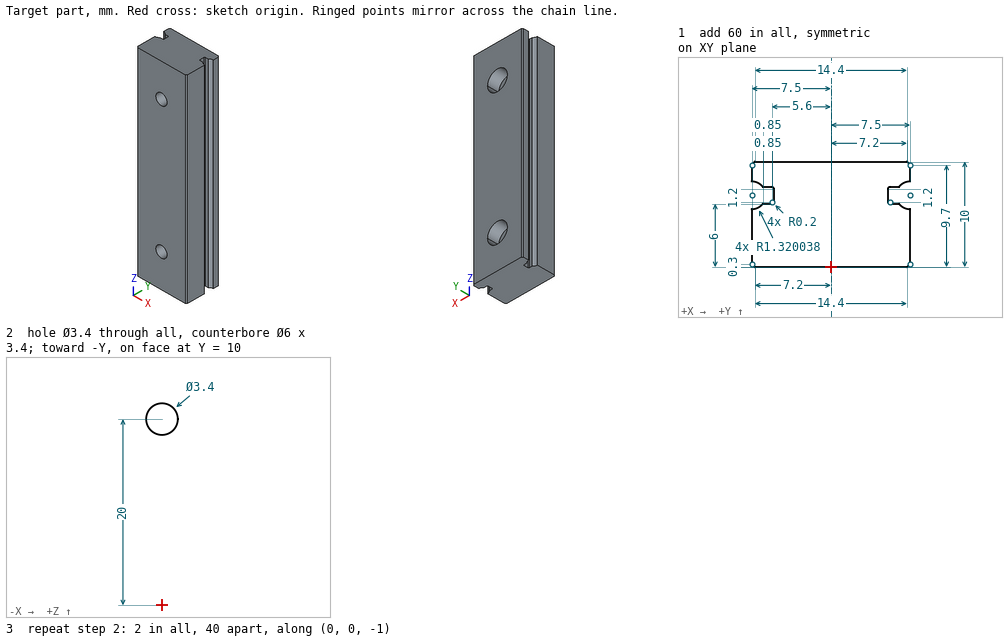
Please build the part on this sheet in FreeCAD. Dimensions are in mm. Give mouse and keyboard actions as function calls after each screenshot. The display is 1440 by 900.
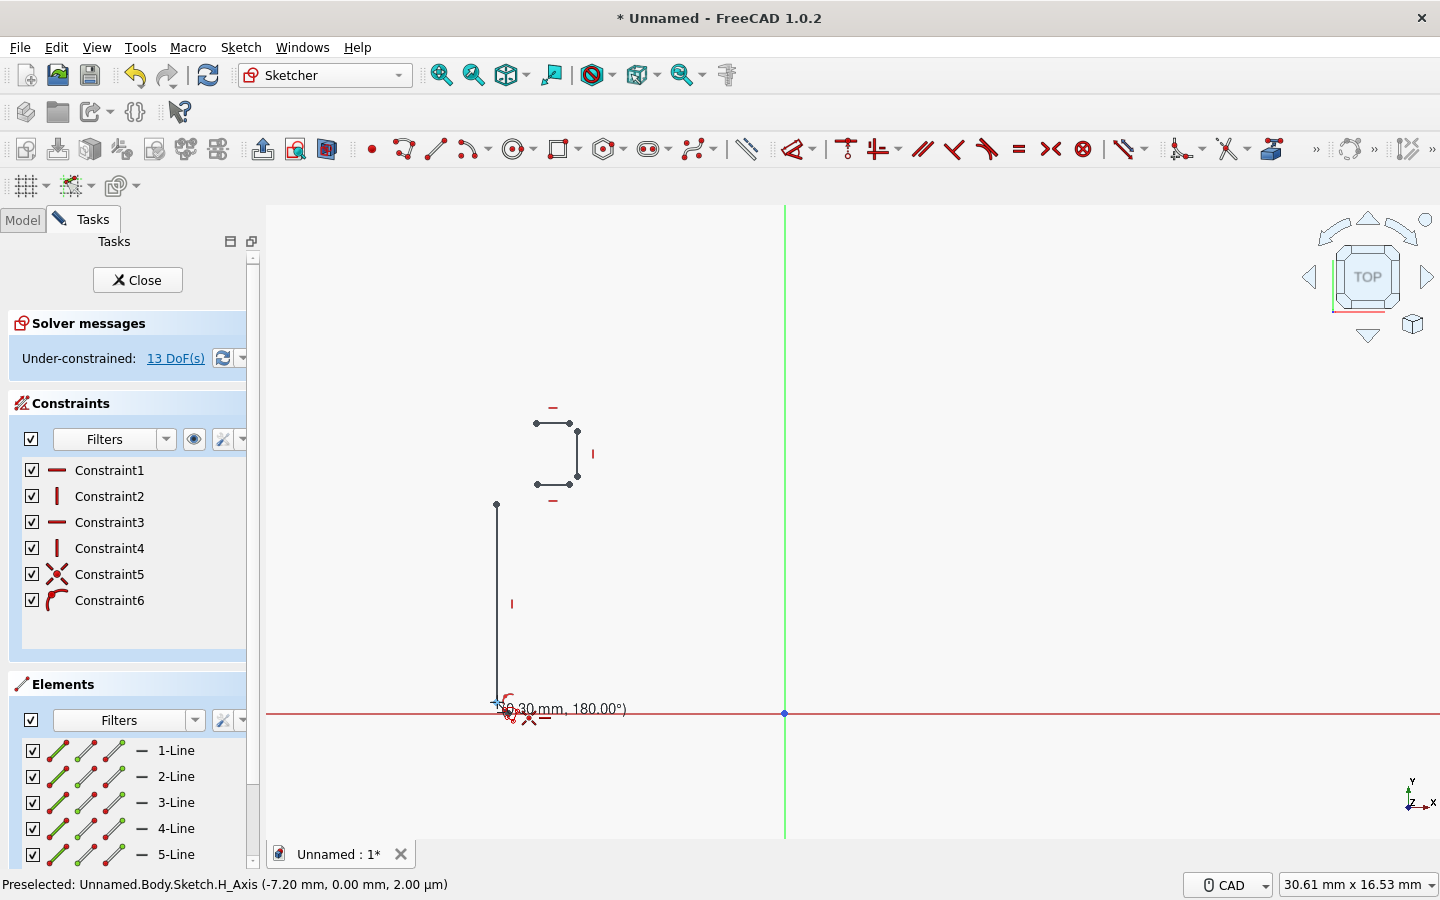
click(1061, 705)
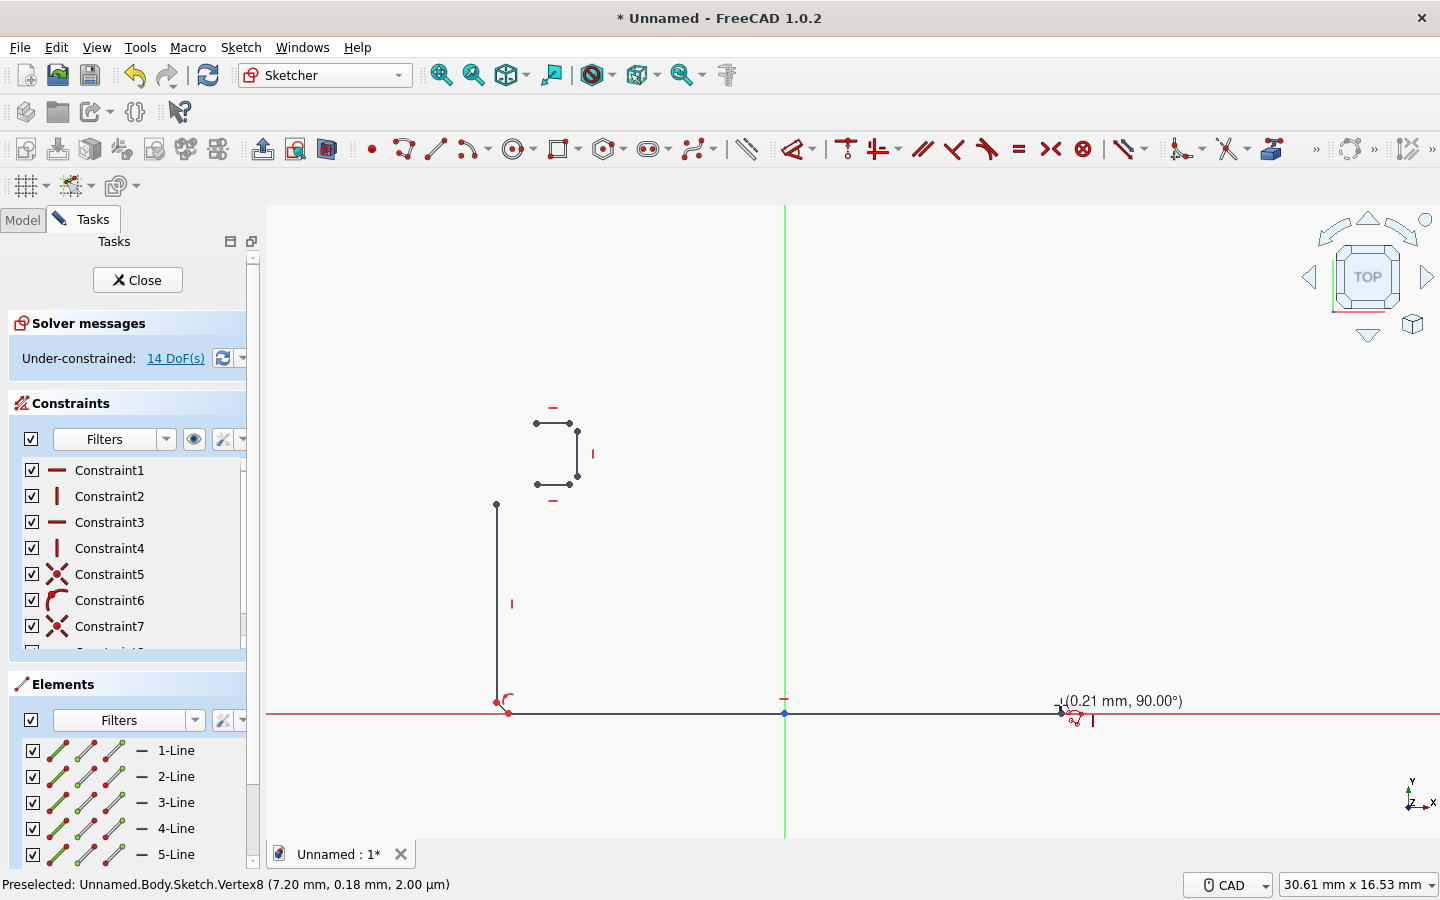
scroll(1072, 702, up, 2)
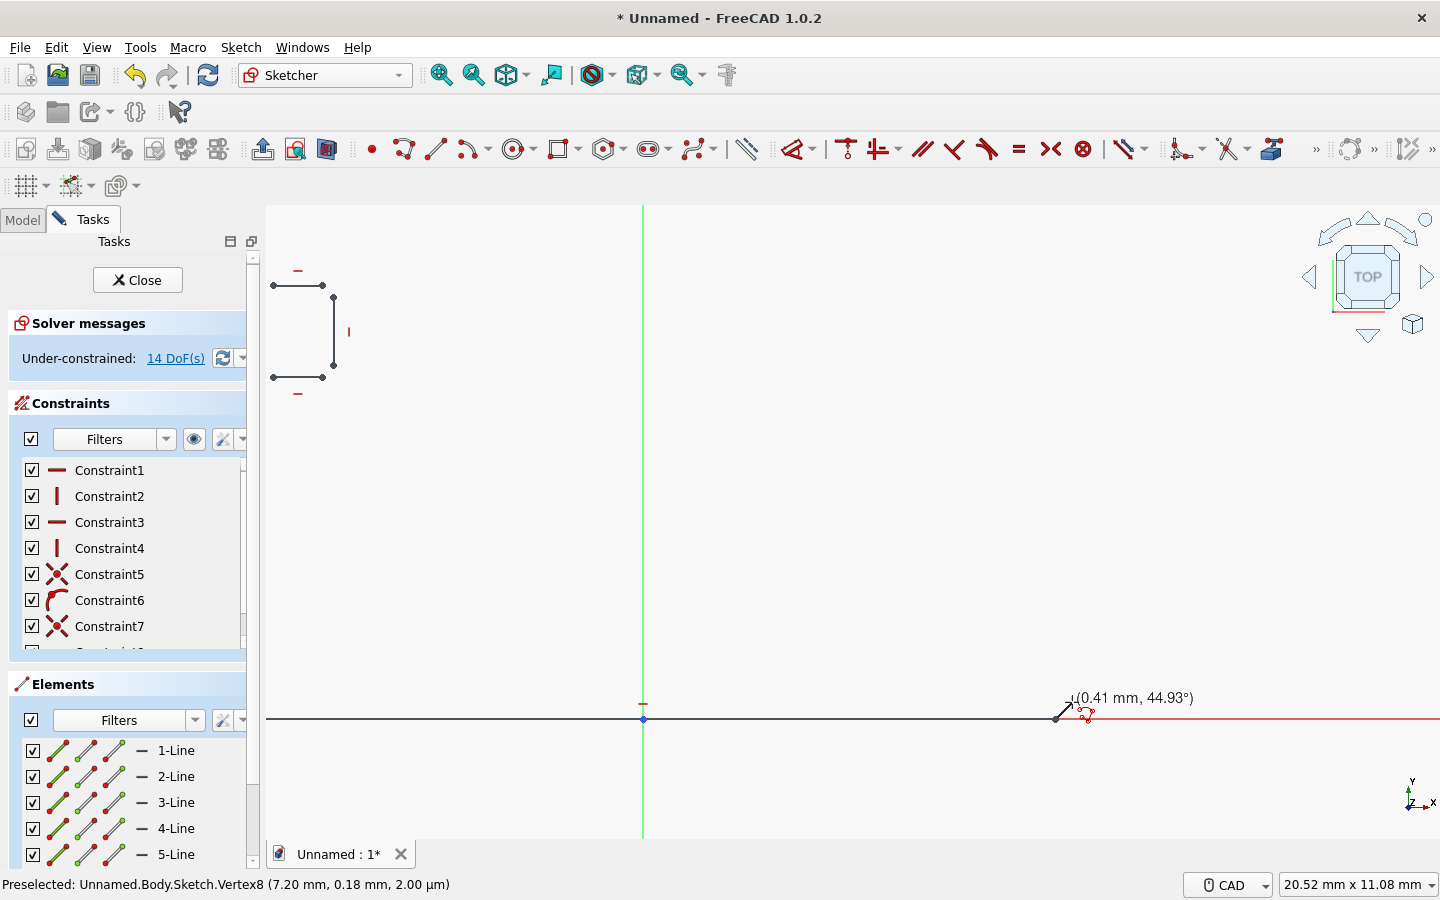
click(1072, 702)
click(1072, 406)
right_click(1072, 406)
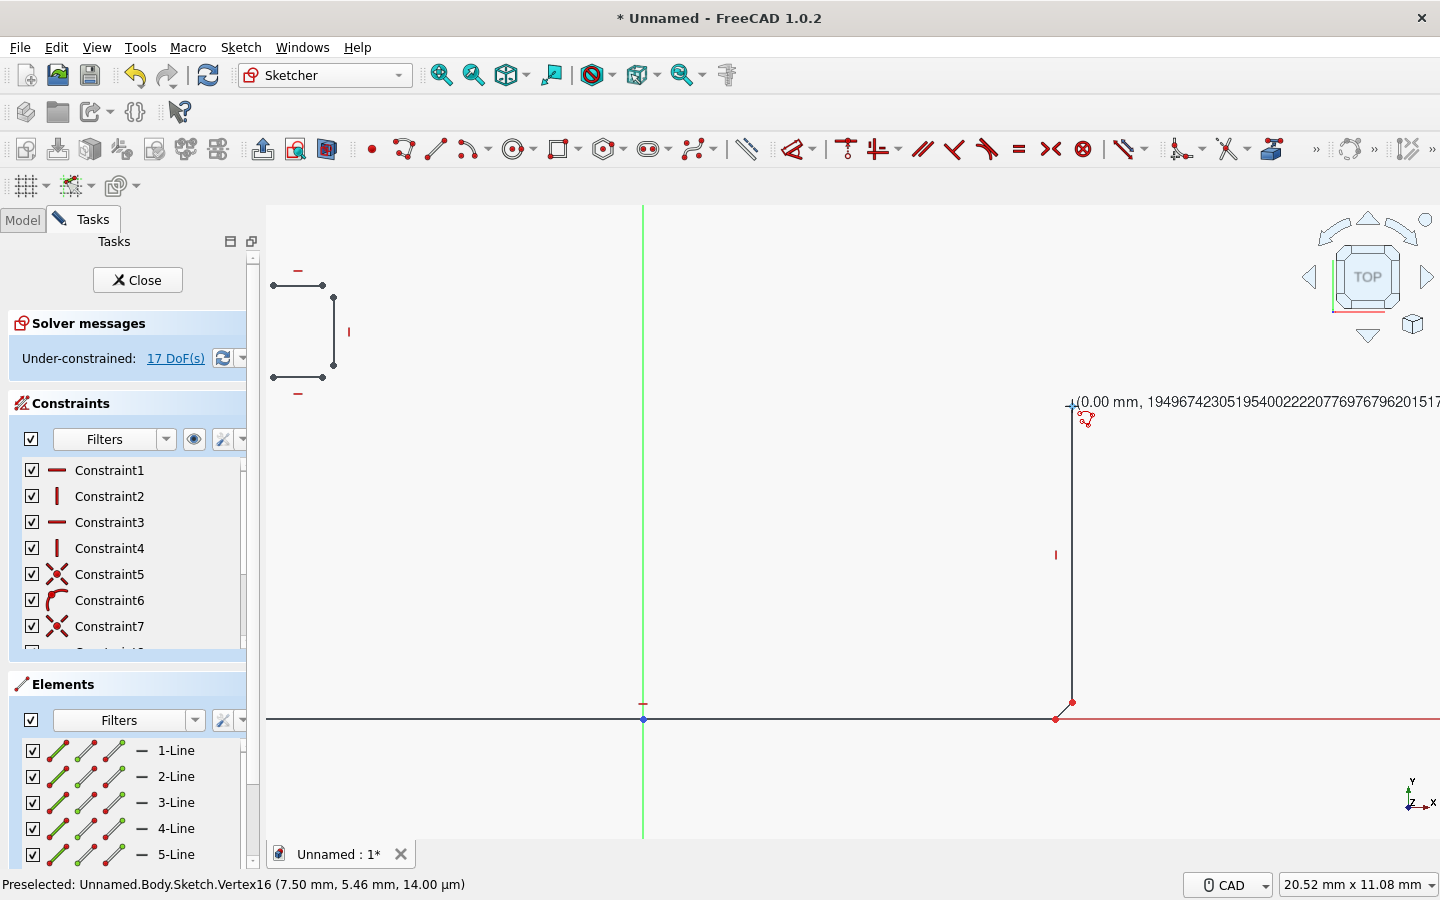
click(436, 150)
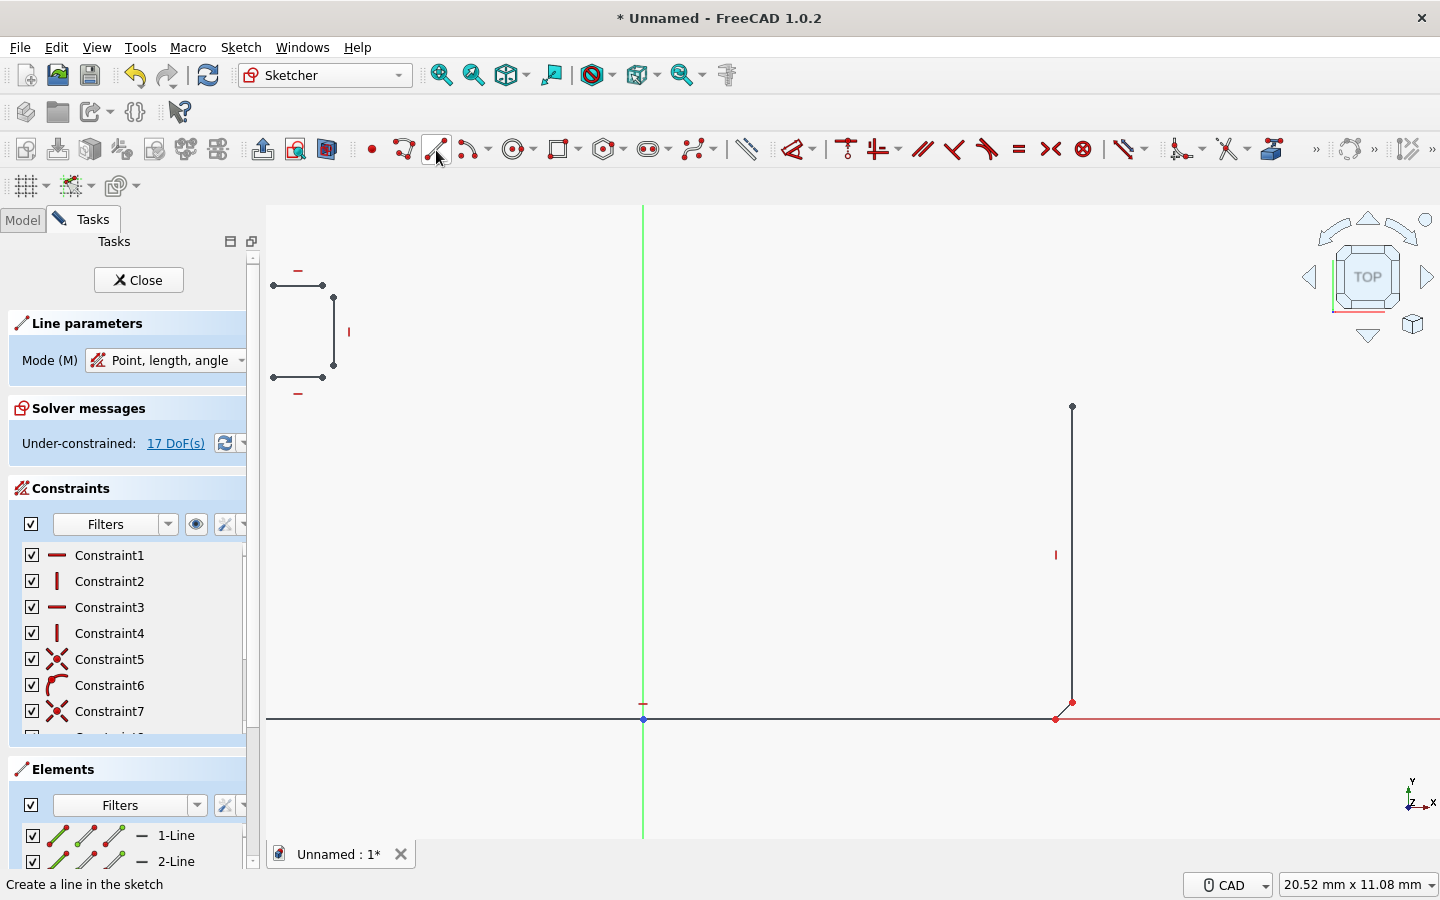
click(1012, 376)
click(963, 376)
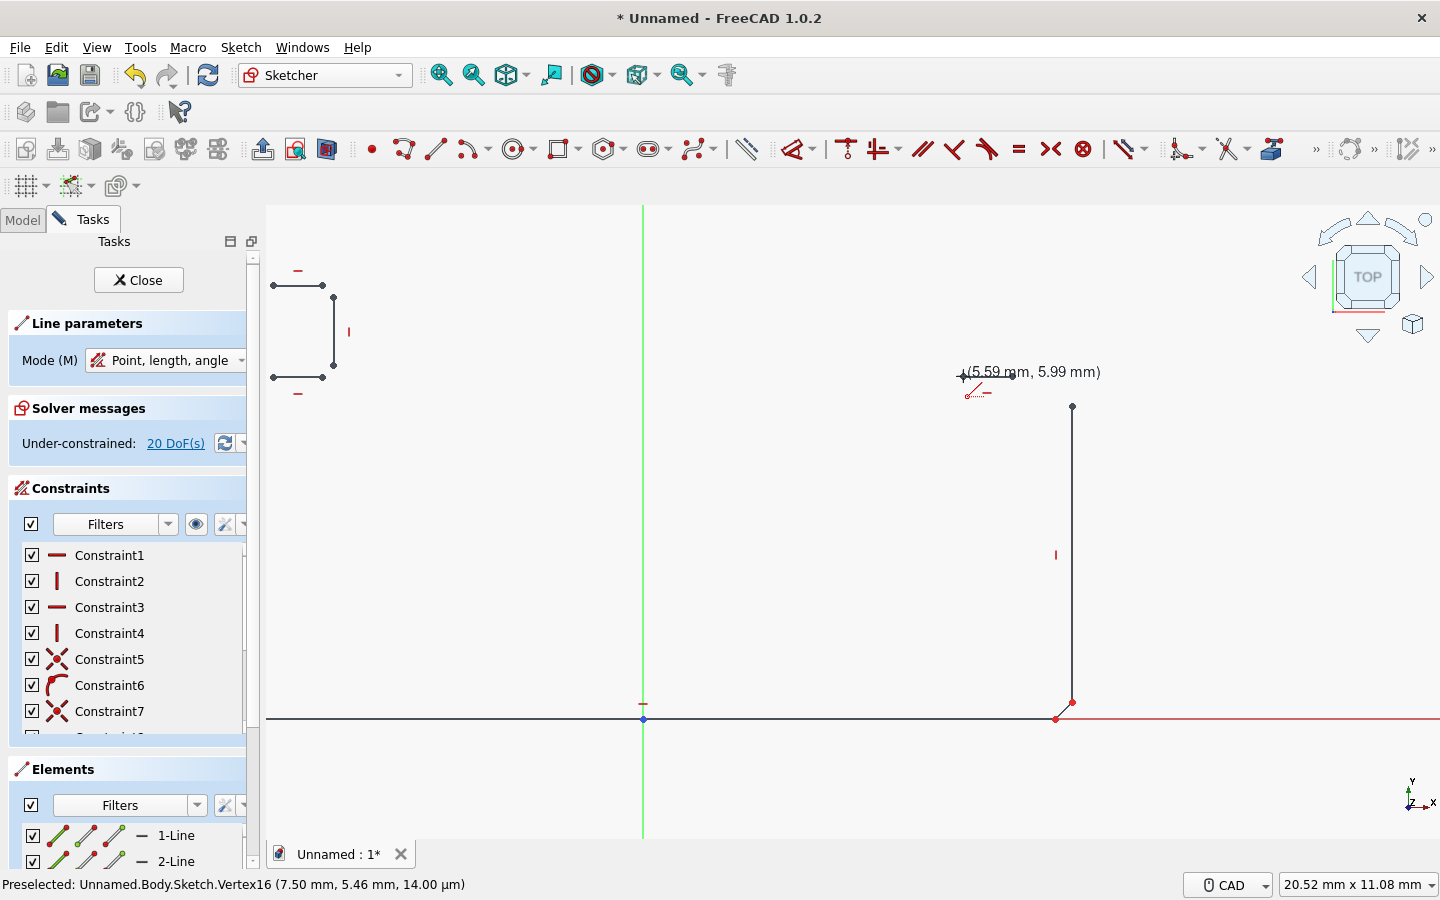
click(952, 365)
click(952, 296)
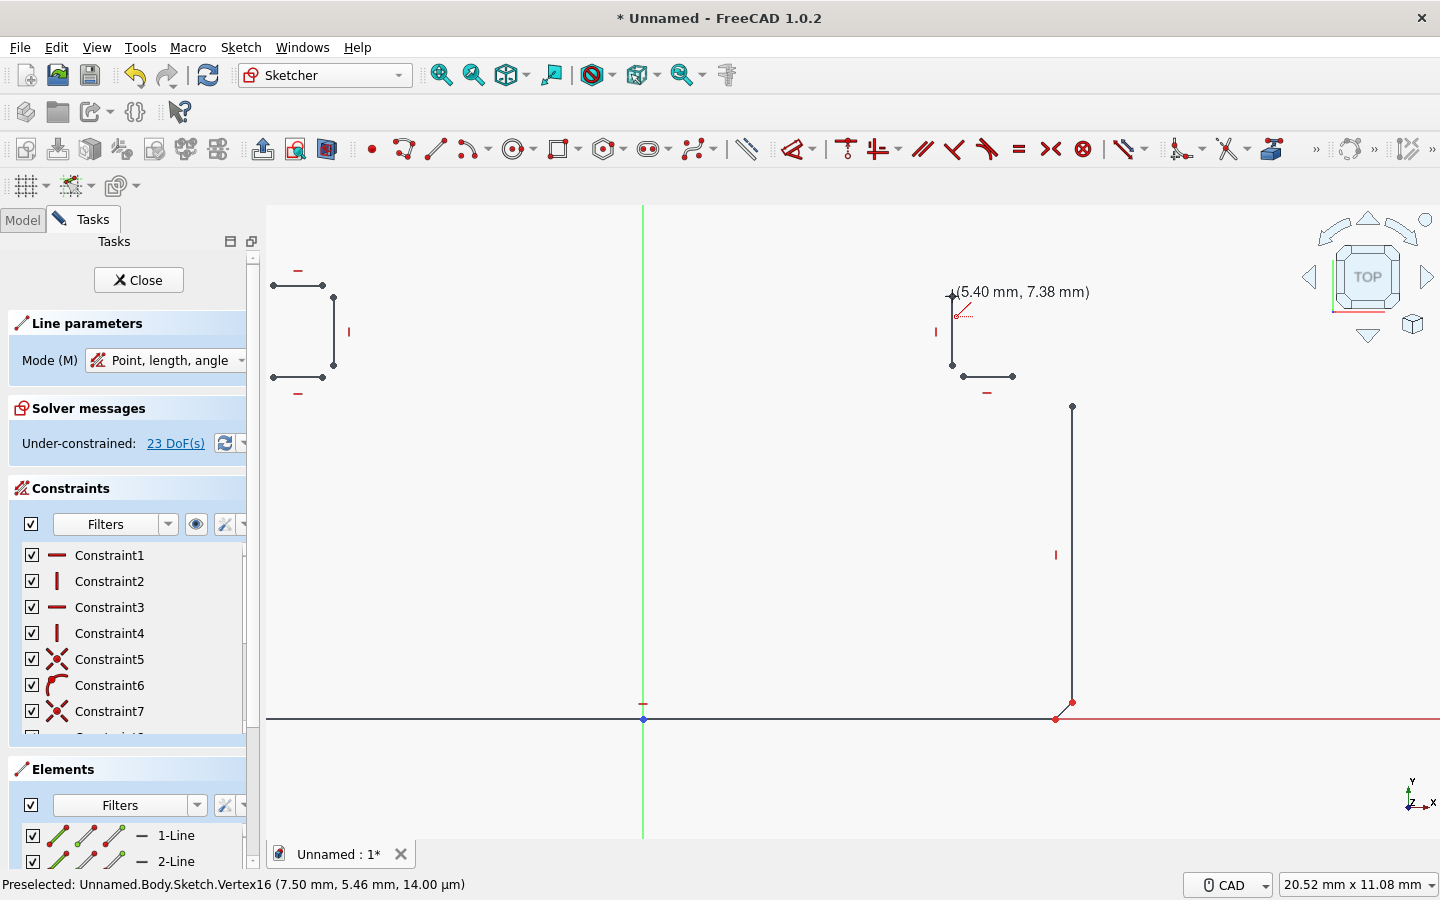
click(963, 285)
click(1012, 285)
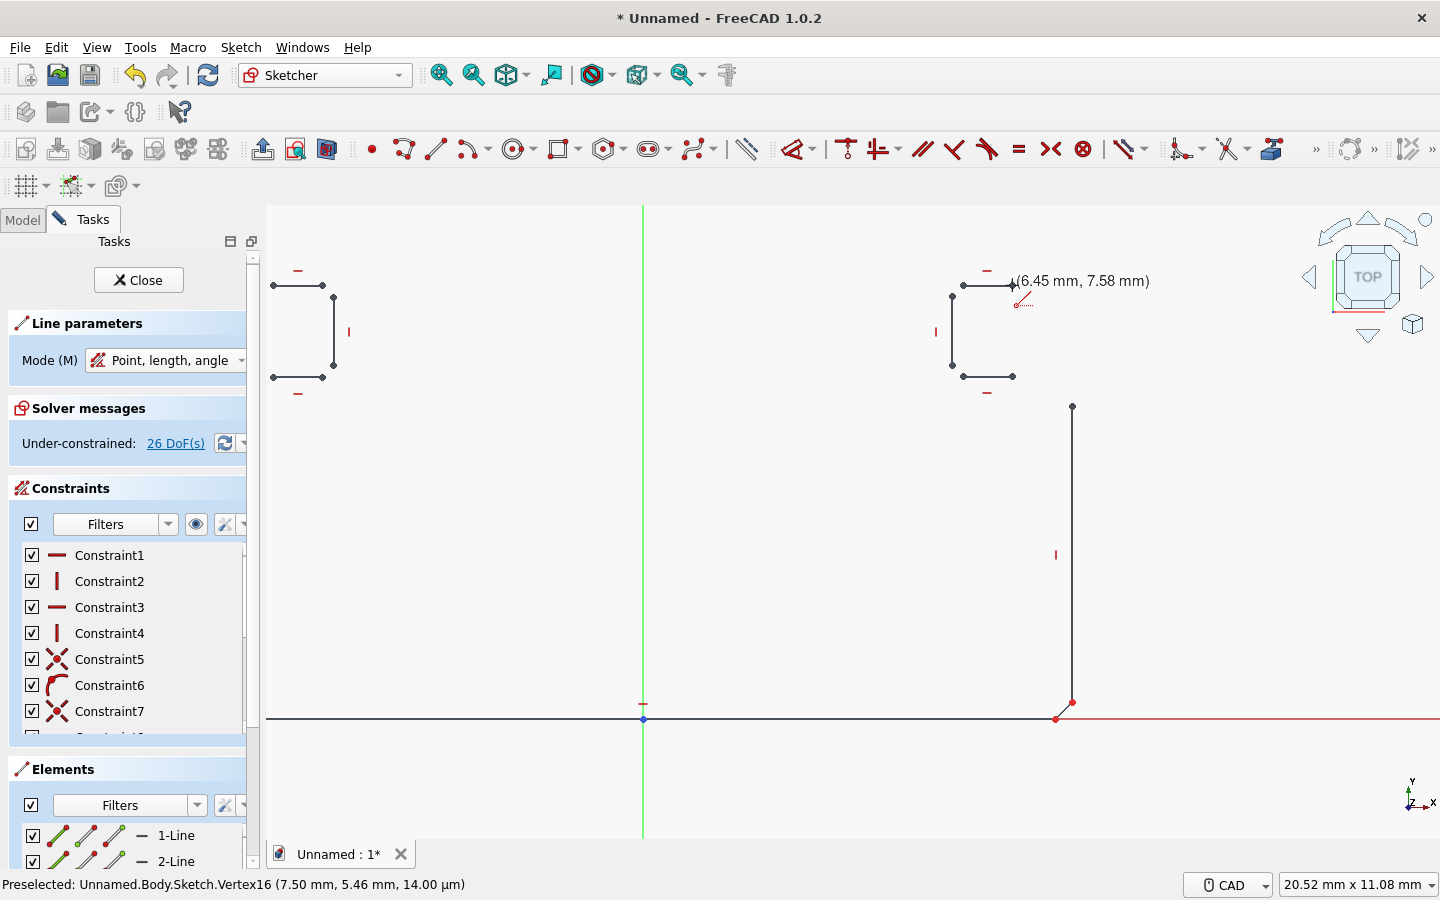
click(404, 150)